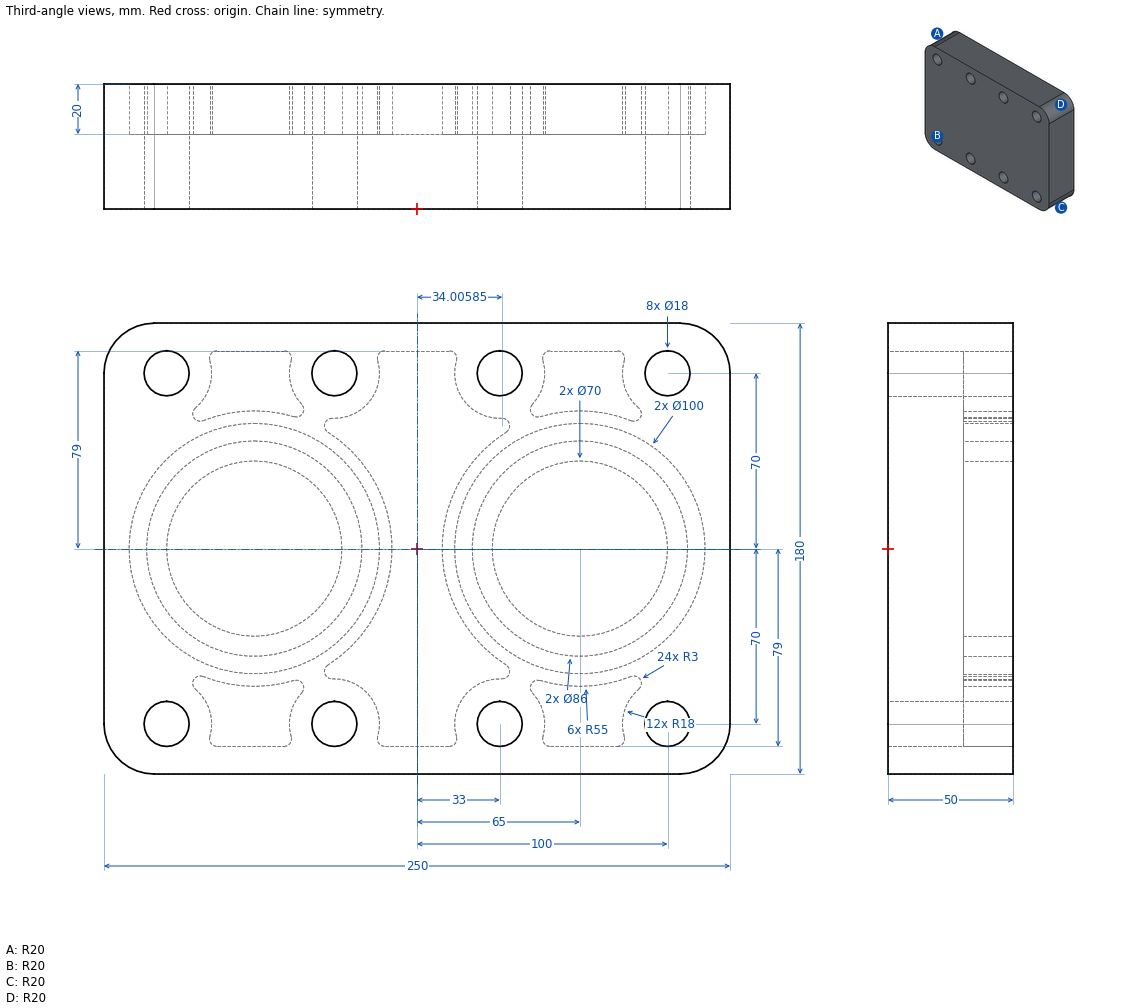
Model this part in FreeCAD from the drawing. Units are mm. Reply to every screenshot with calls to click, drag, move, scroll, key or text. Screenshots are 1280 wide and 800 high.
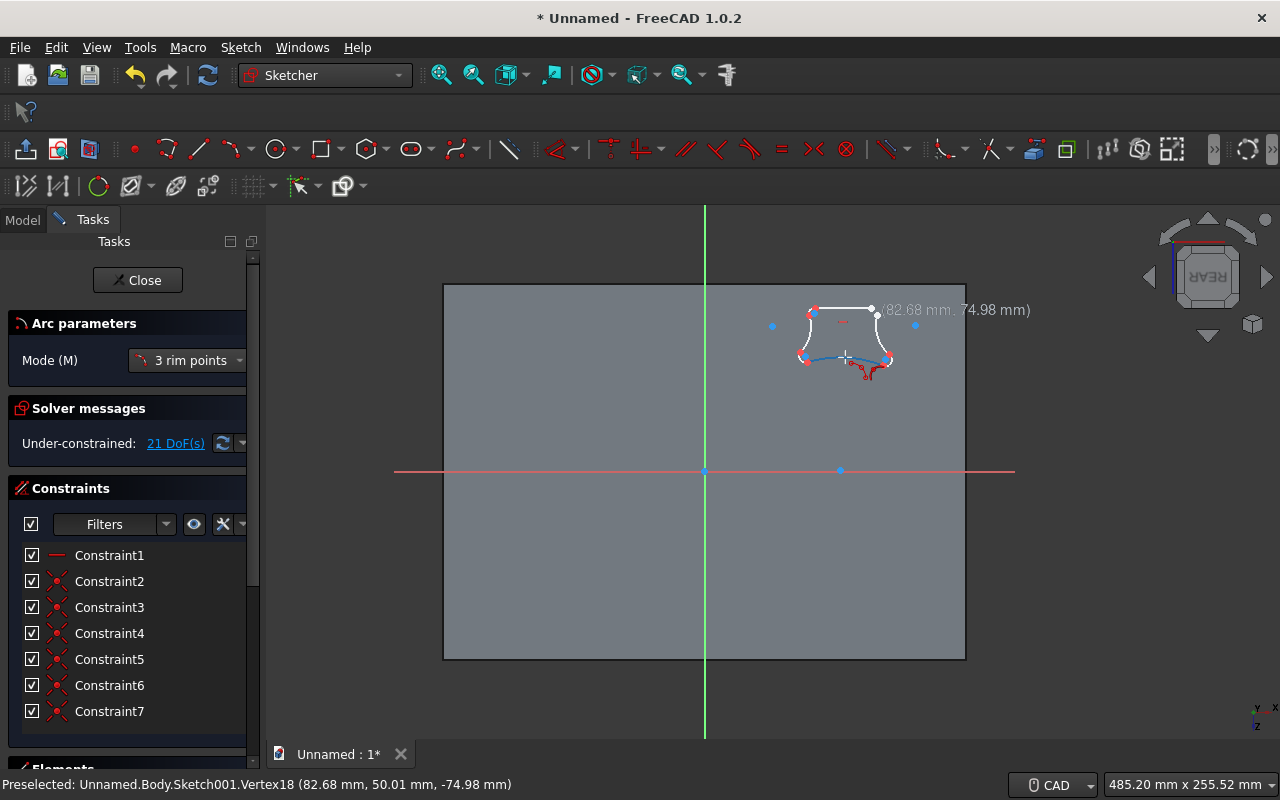
scroll(872, 307, up, 3)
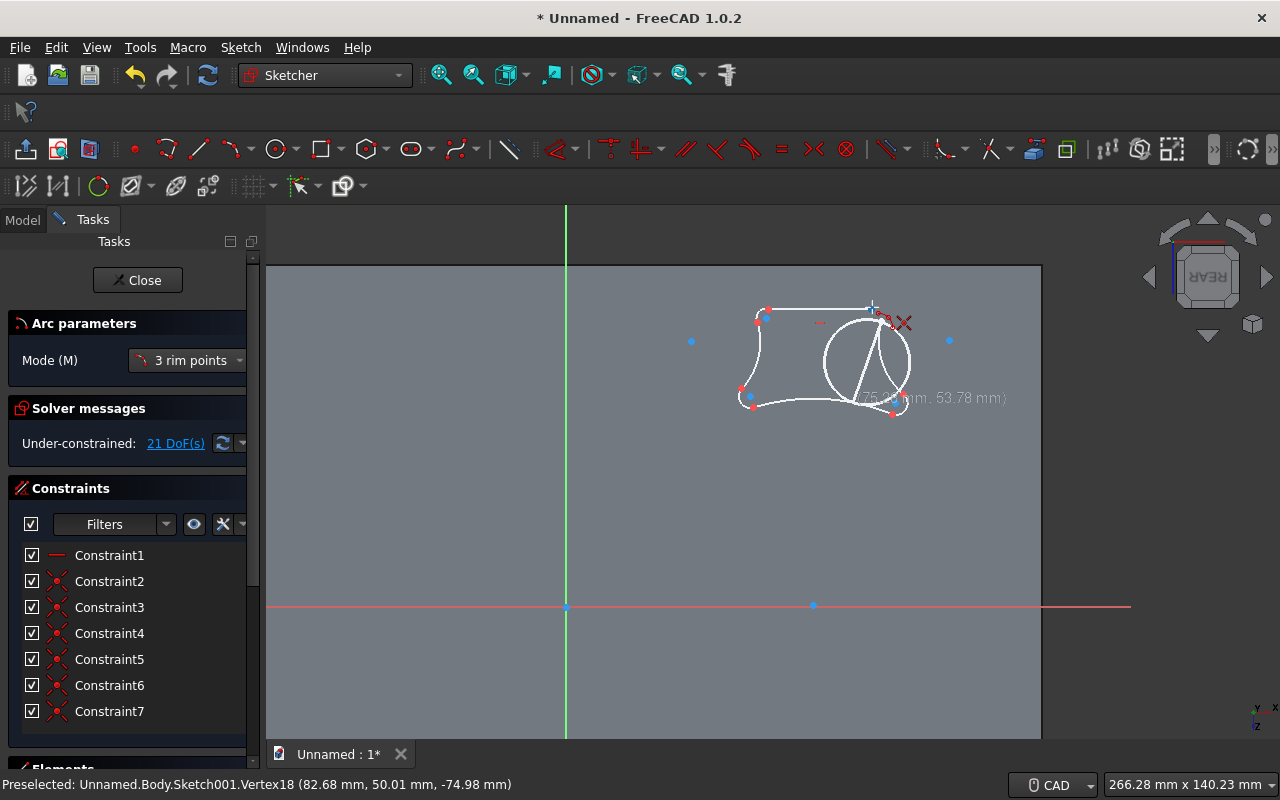
click(871, 309)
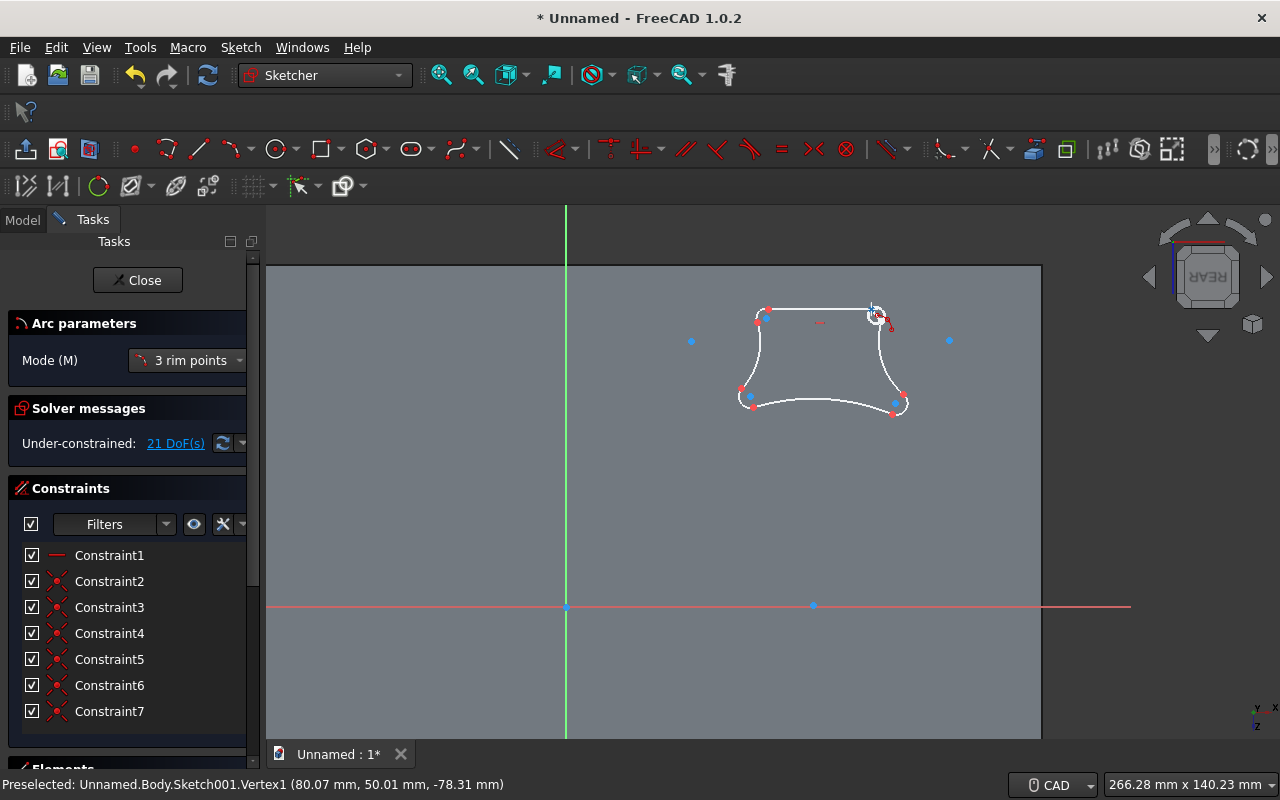
scroll(880, 311, up, 7)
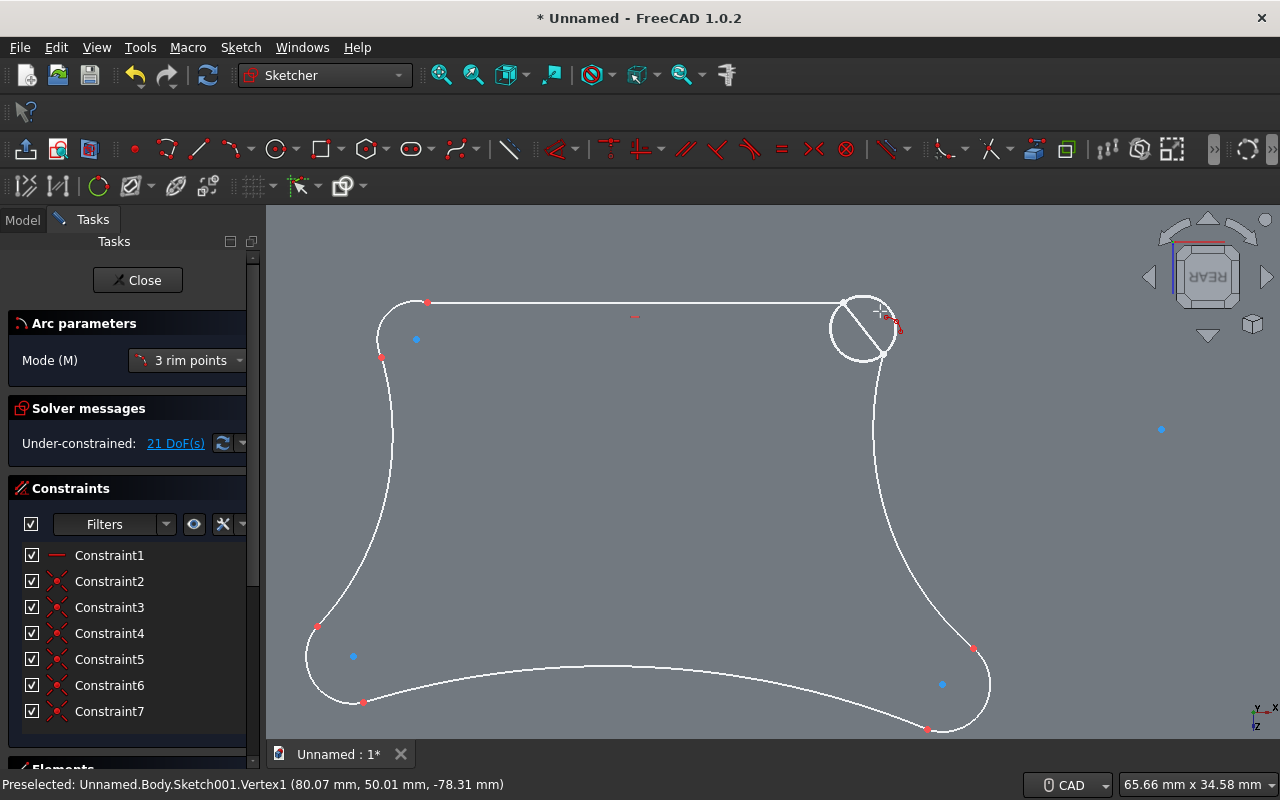
click(877, 311)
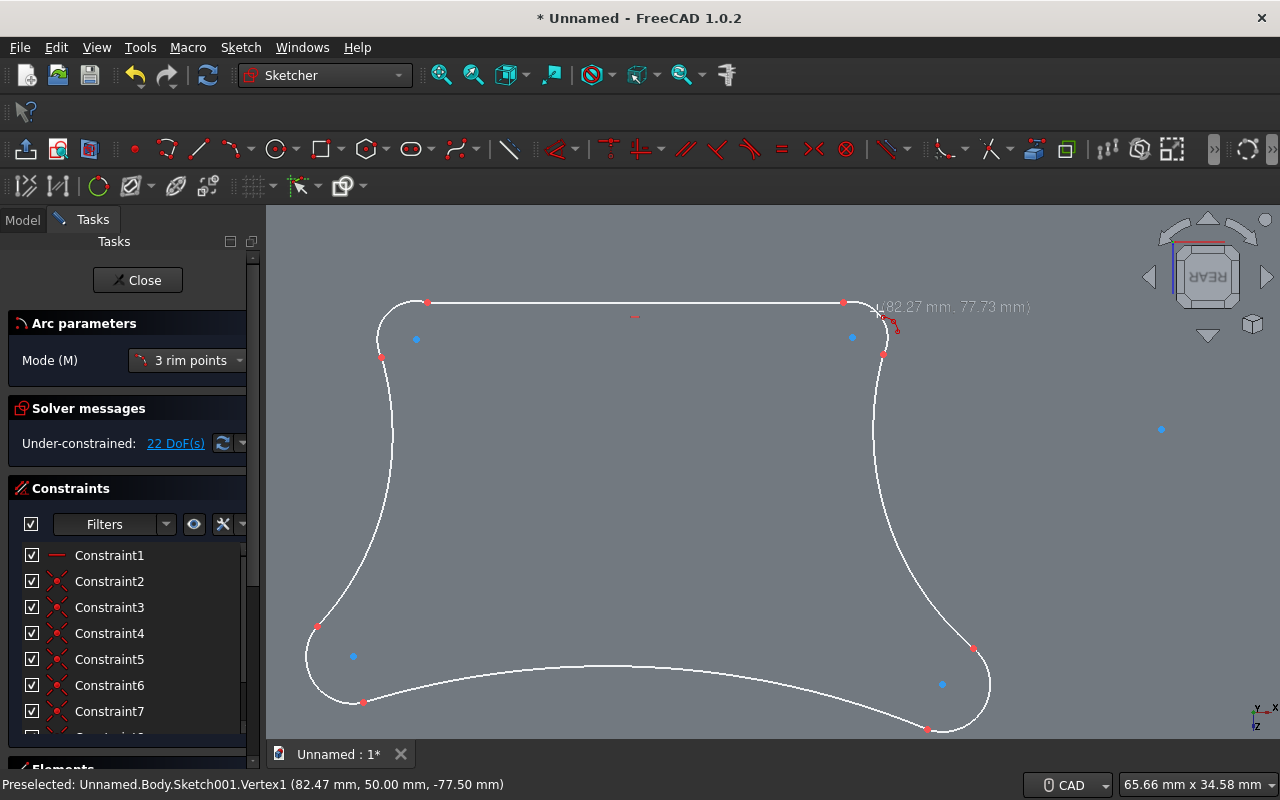
click(200, 150)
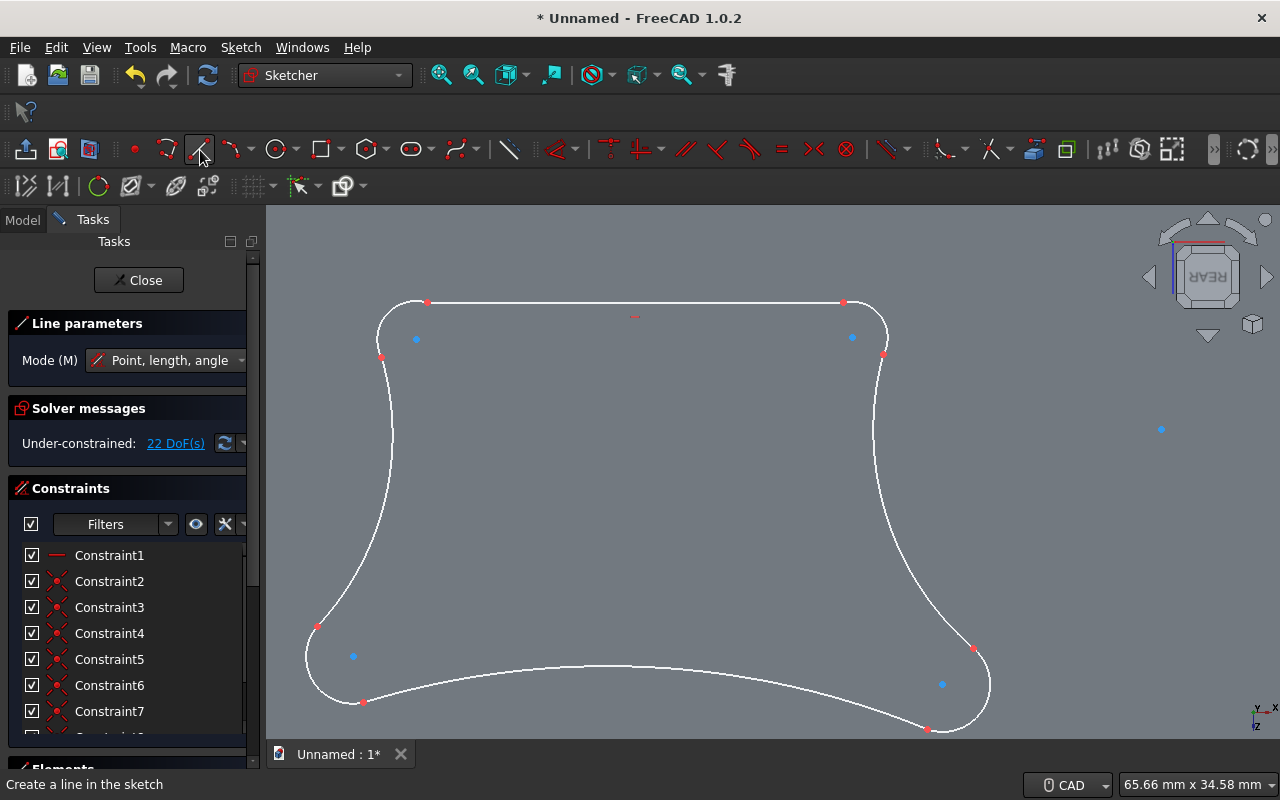
scroll(876, 309, down, 10)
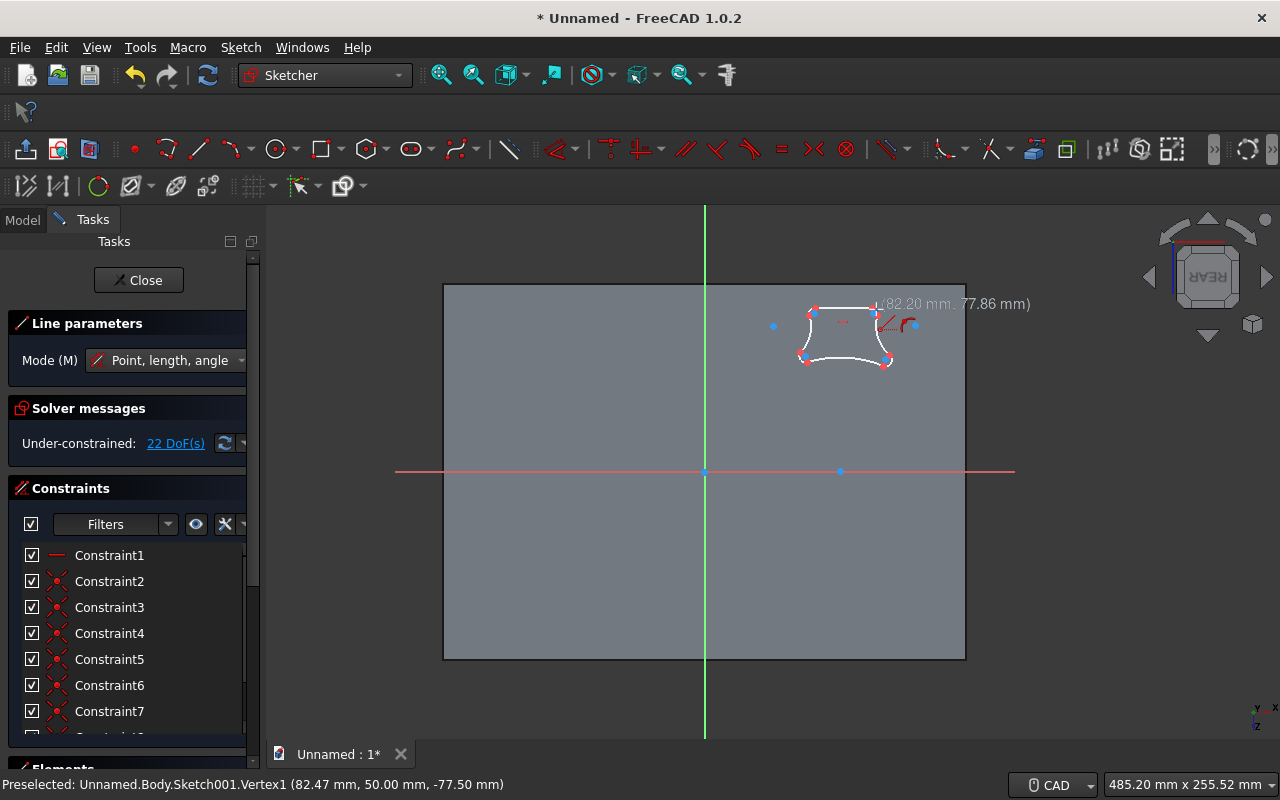
click(678, 637)
click(732, 637)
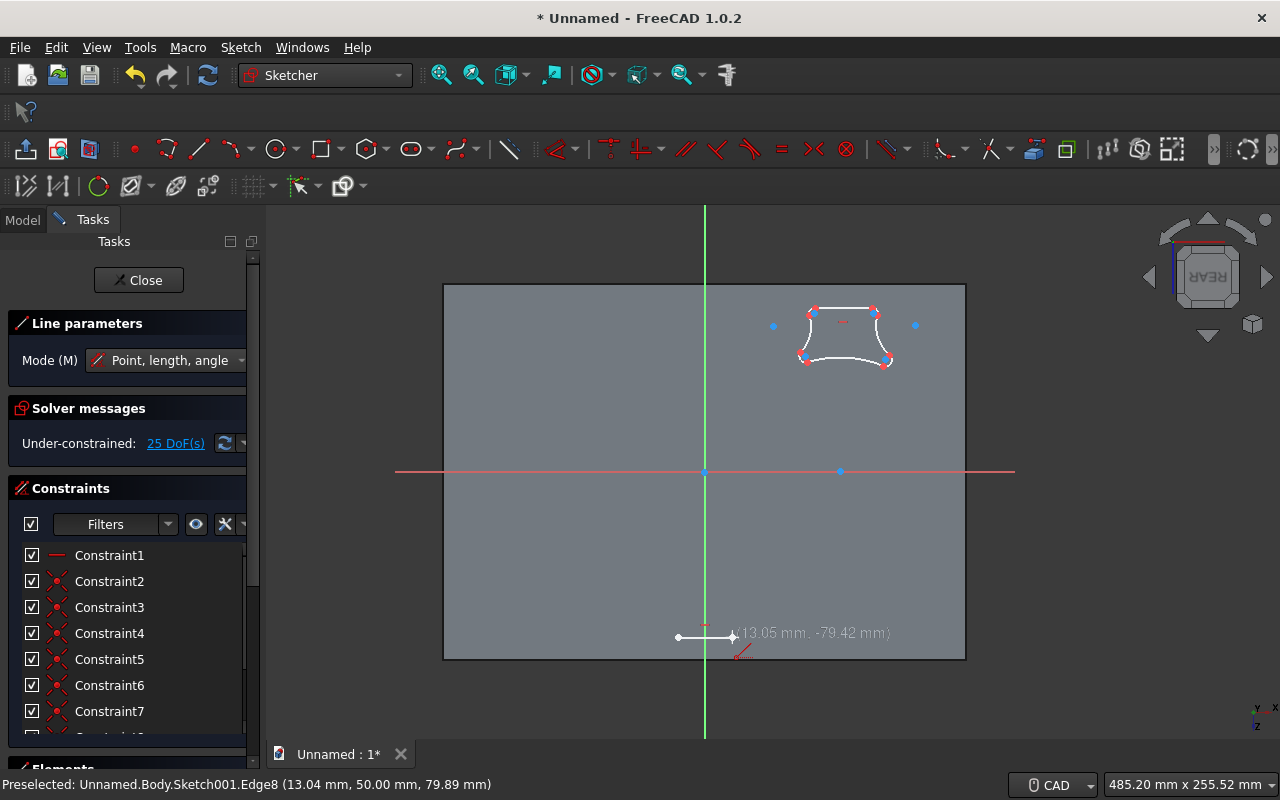
click(732, 307)
click(678, 307)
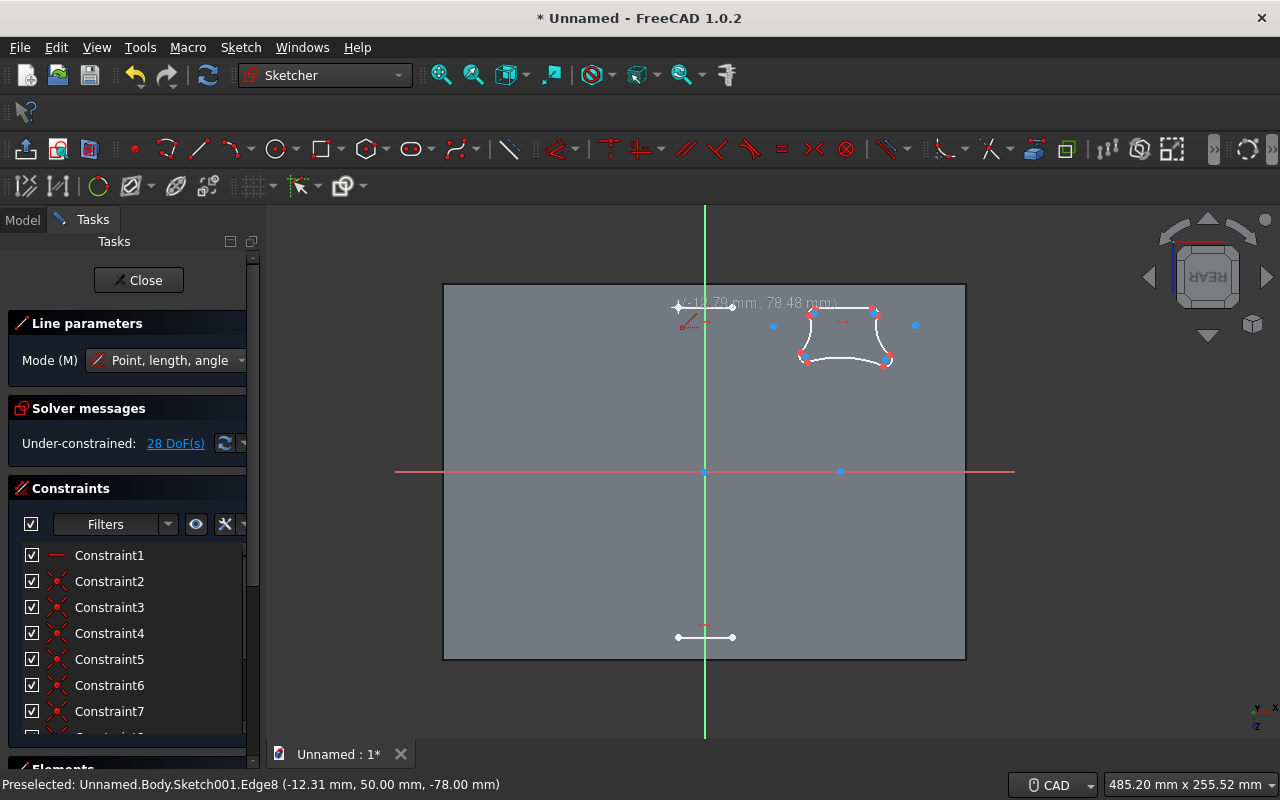
click(232, 150)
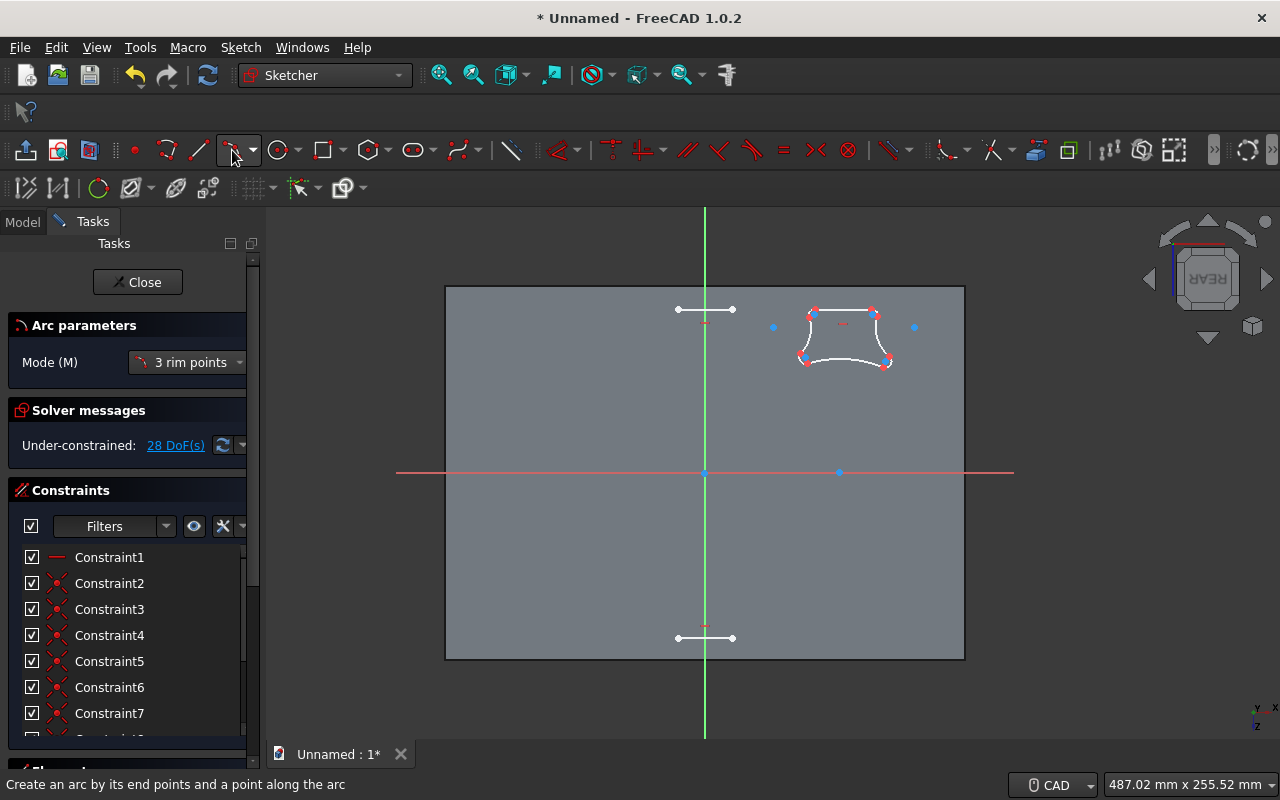
click(732, 638)